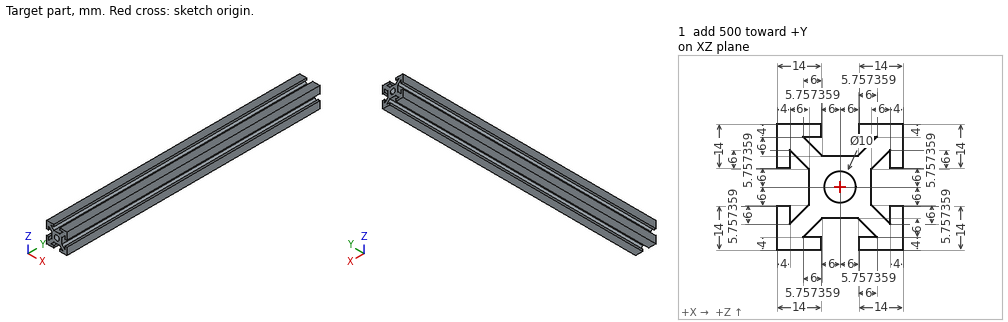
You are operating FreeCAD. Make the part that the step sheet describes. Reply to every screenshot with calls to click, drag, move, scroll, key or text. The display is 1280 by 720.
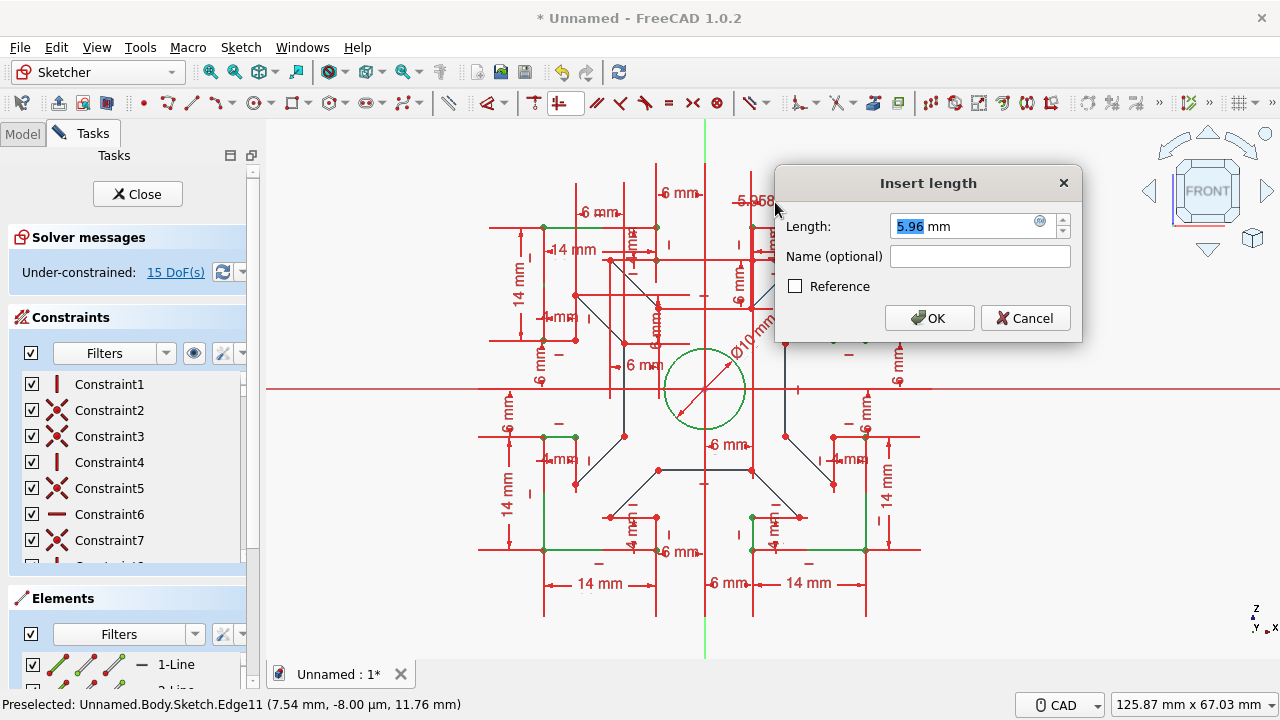
text(6)
key(Return)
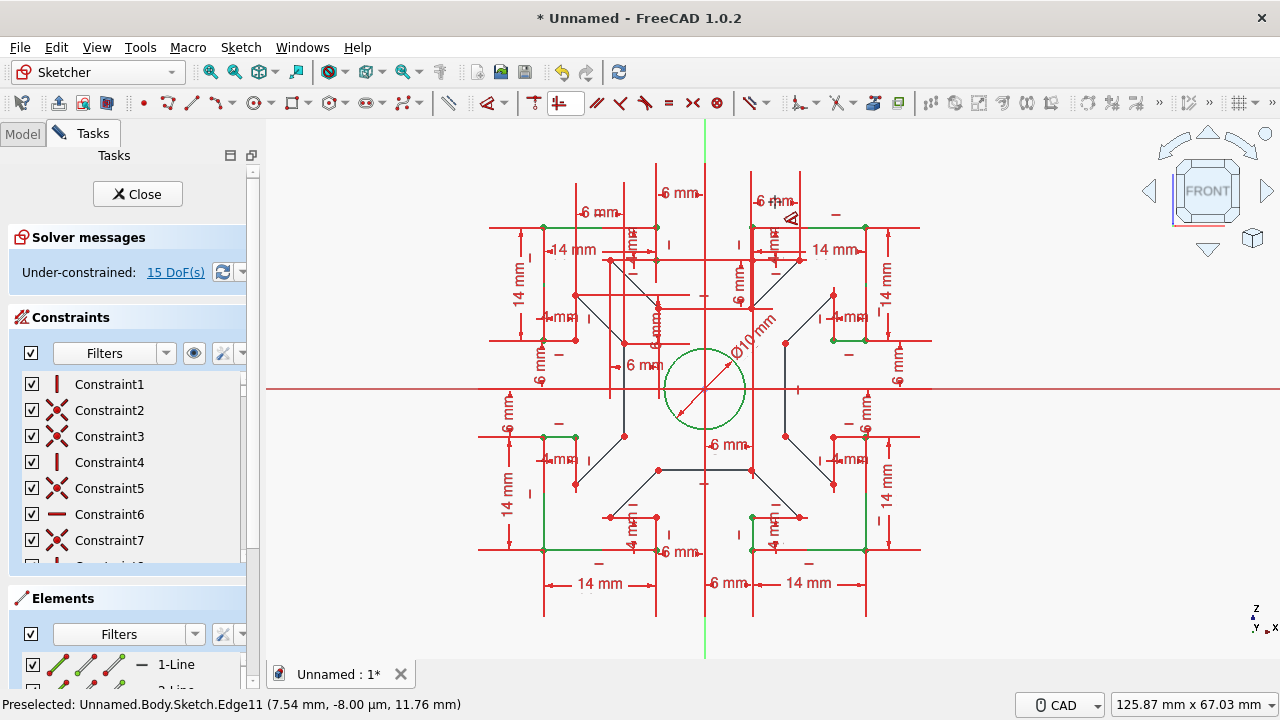
click(819, 310)
click(809, 165)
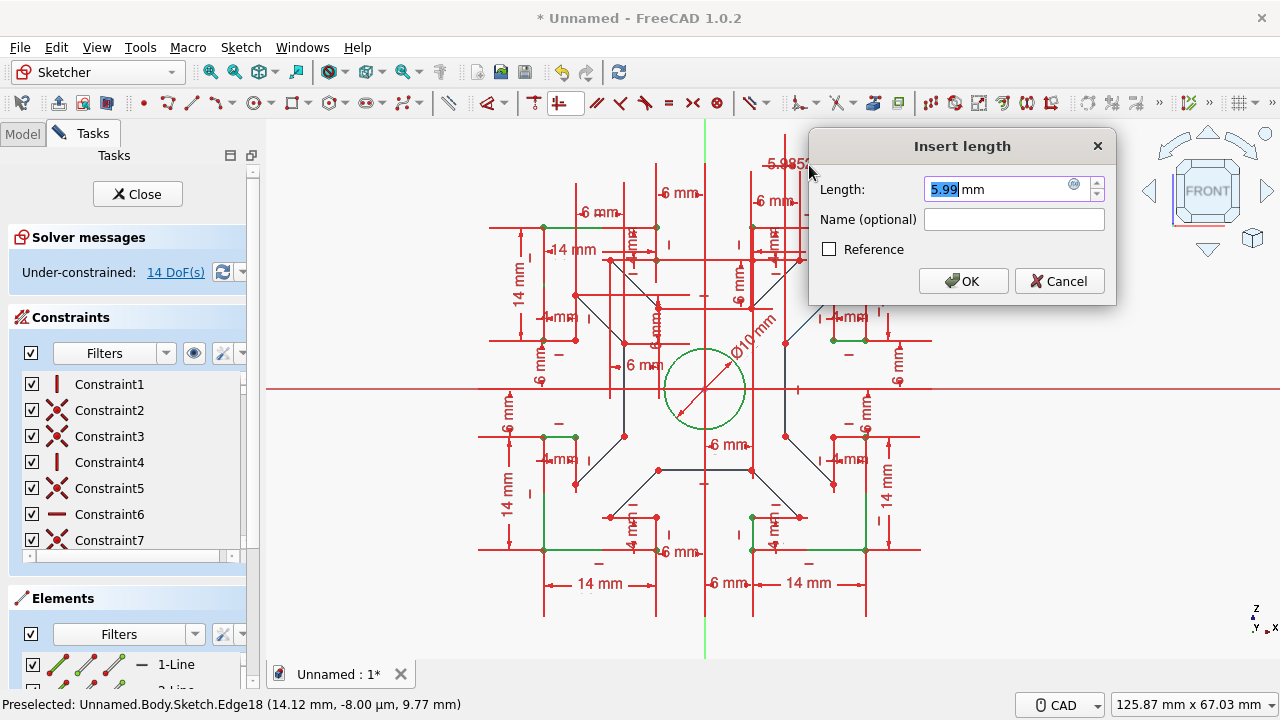
text(6)
key(Return)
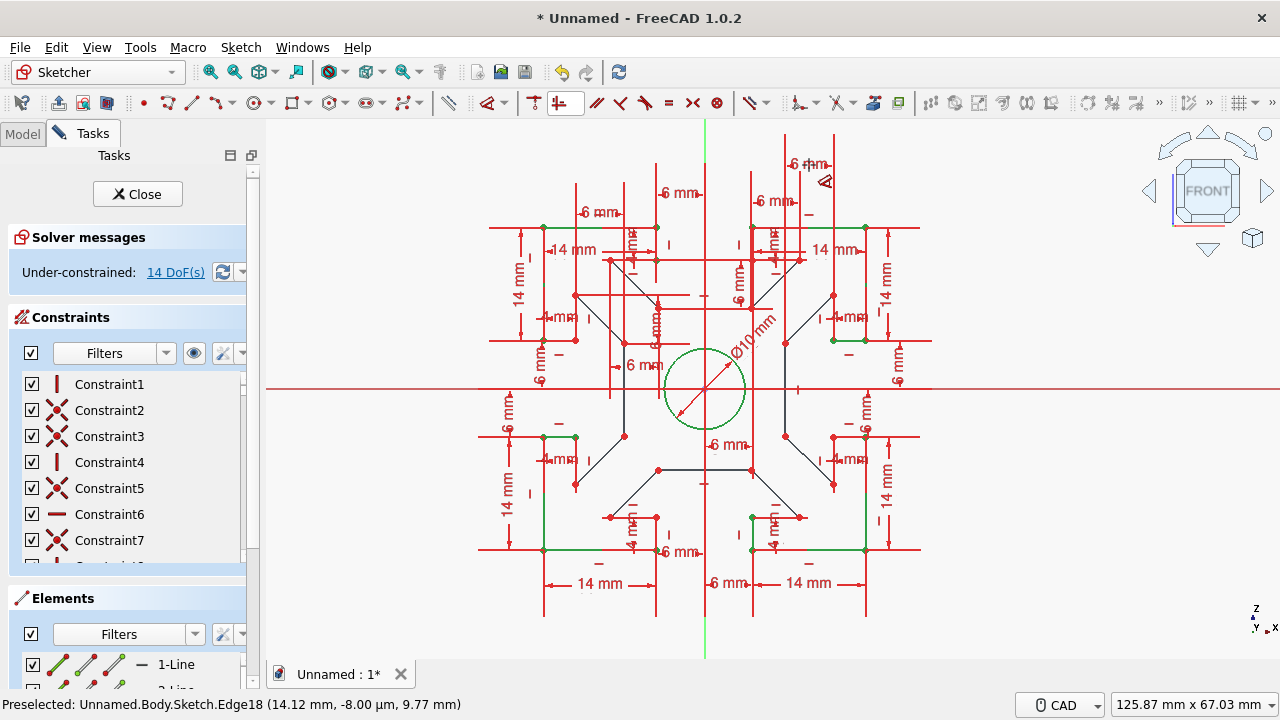
click(819, 310)
click(940, 319)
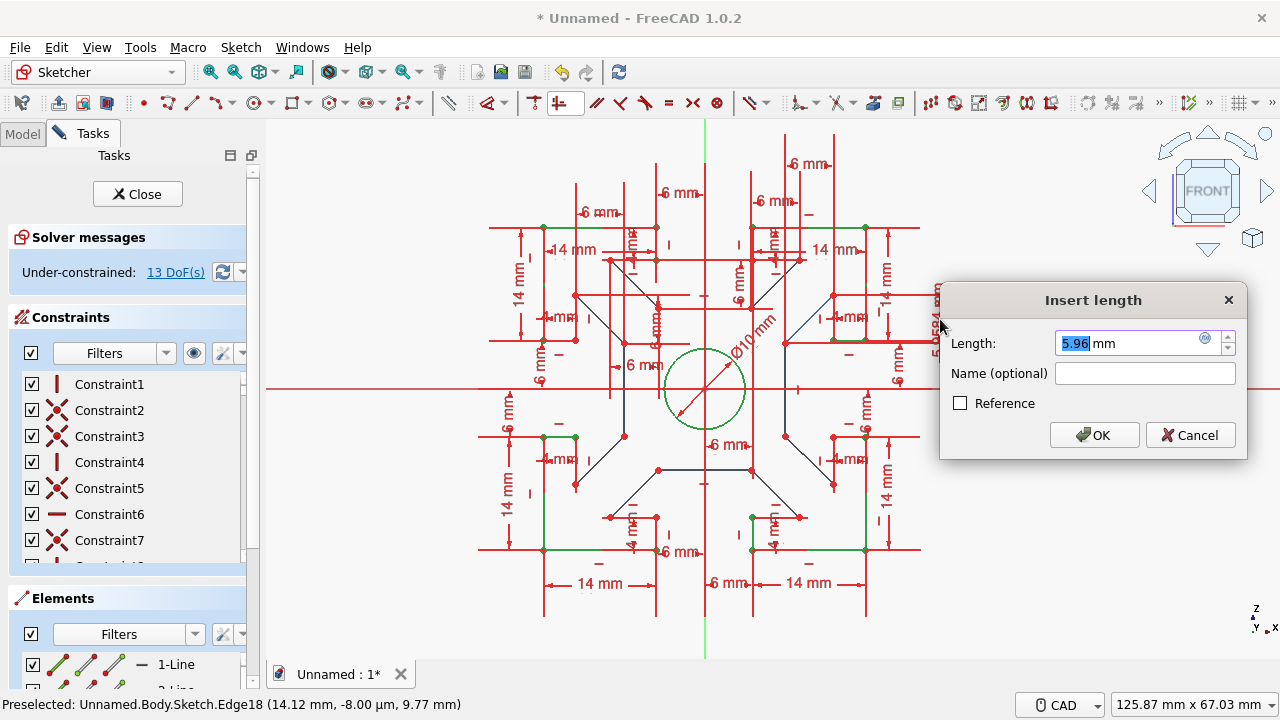
text(6)
key(Return)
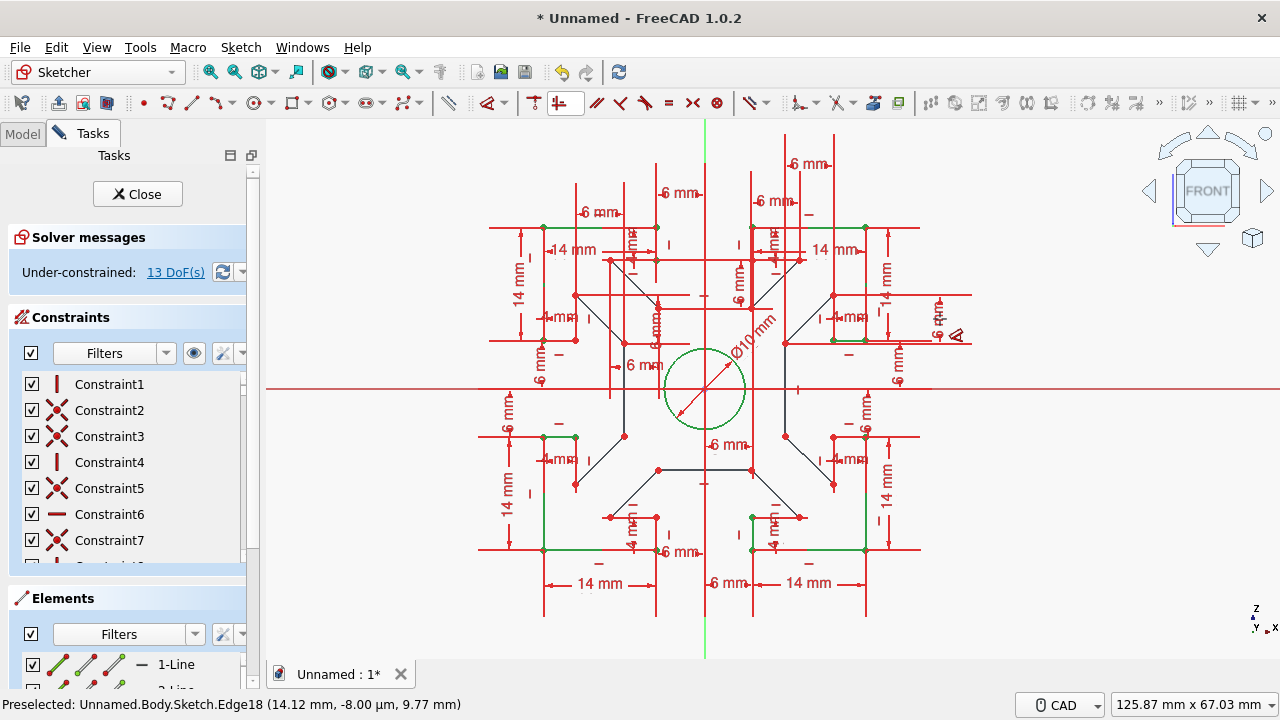
click(800, 451)
click(940, 460)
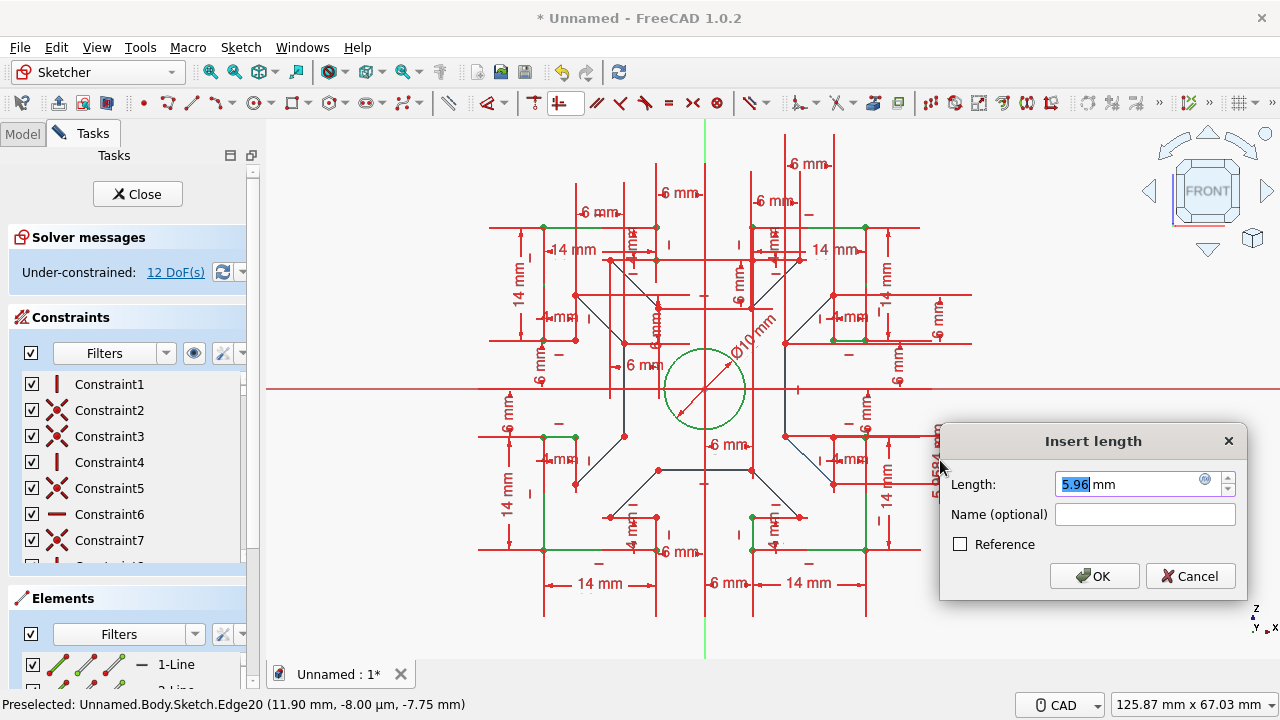
text(6)
key(Return)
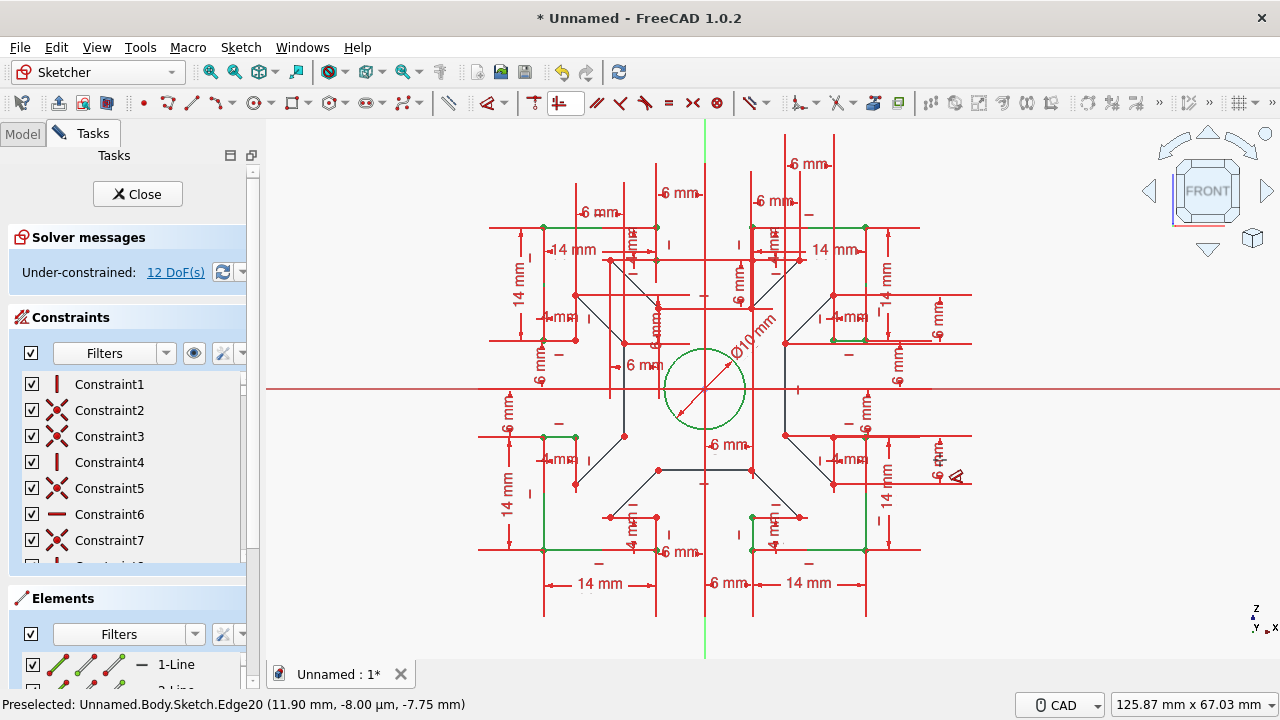
click(785, 504)
click(764, 412)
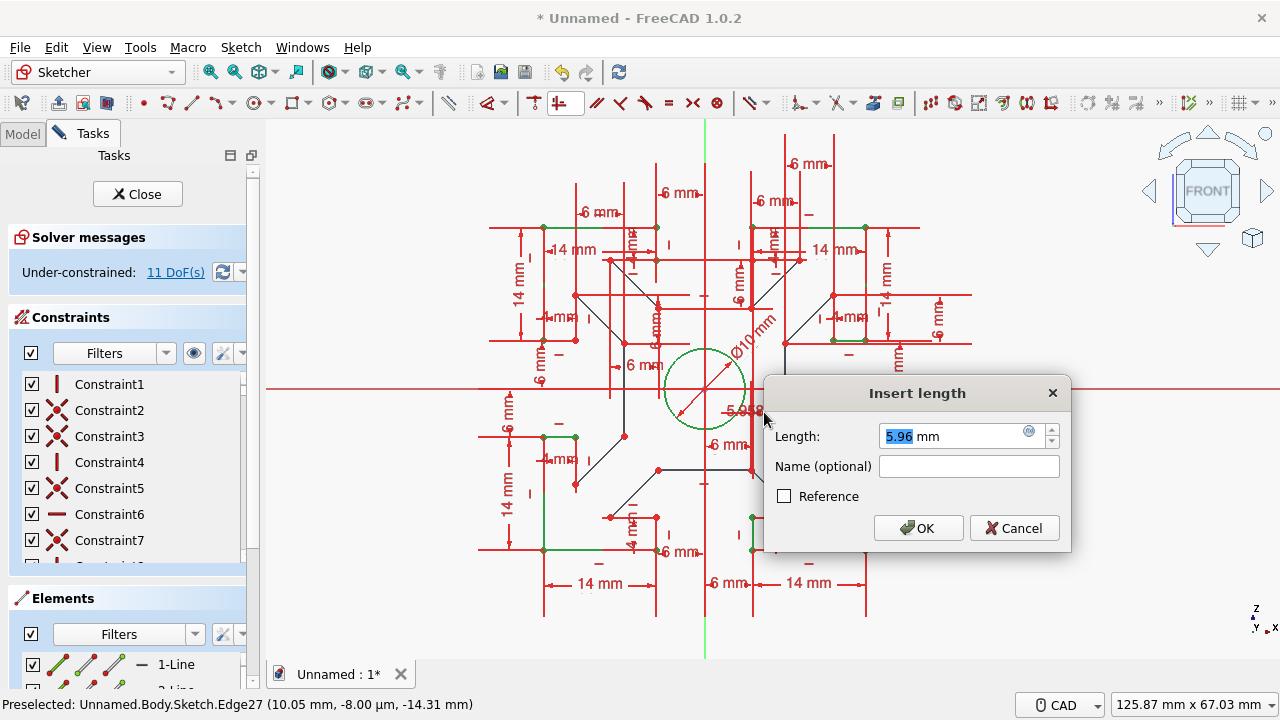
text(6)
key(Return)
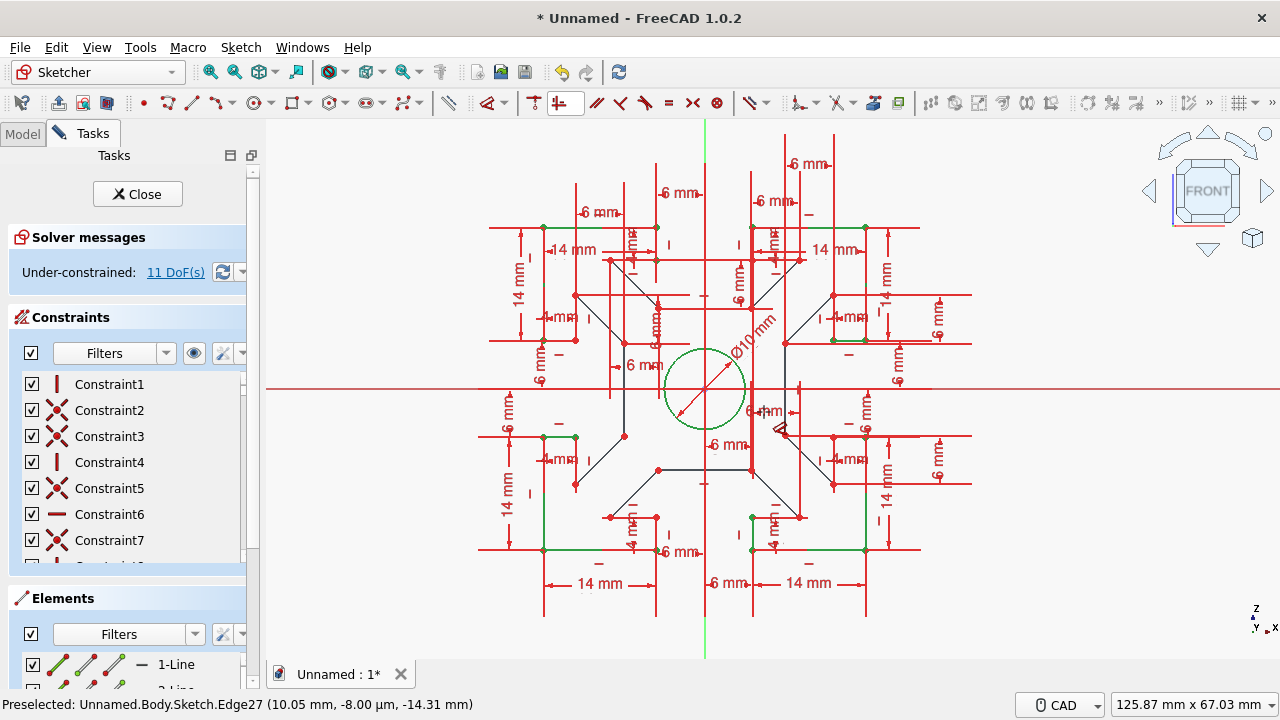
click(785, 504)
click(834, 511)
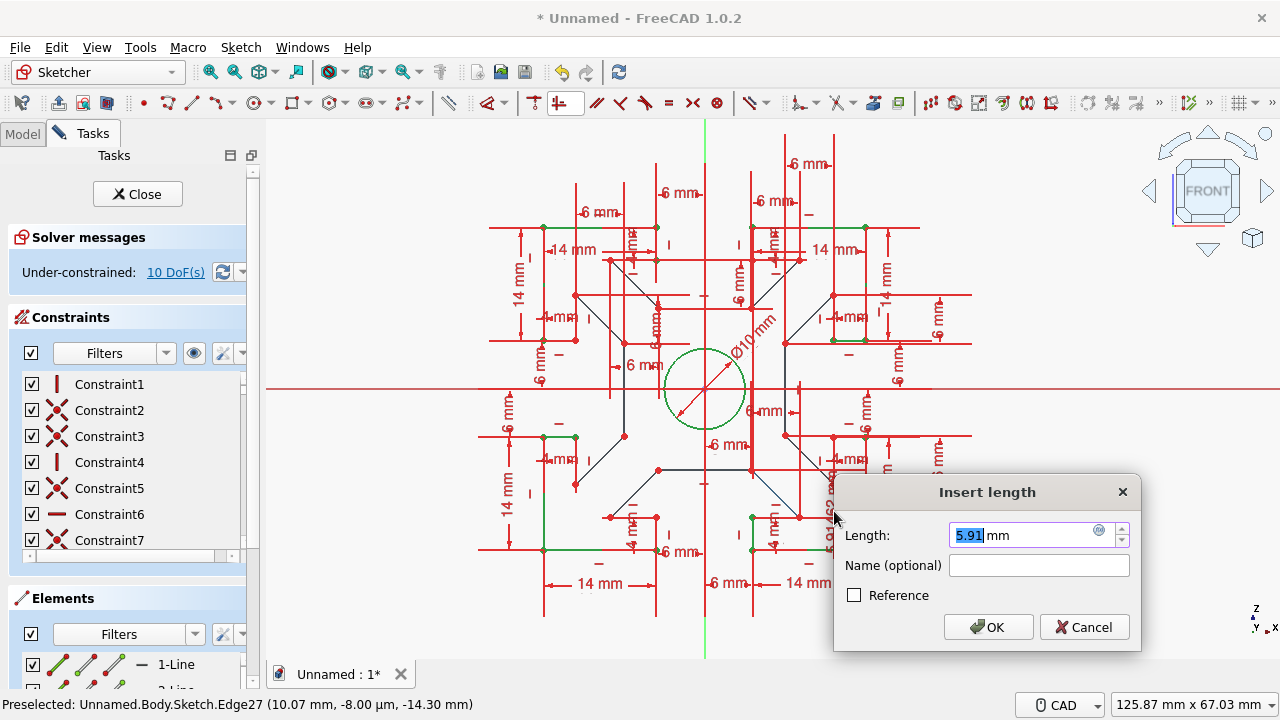
text(6)
key(Return)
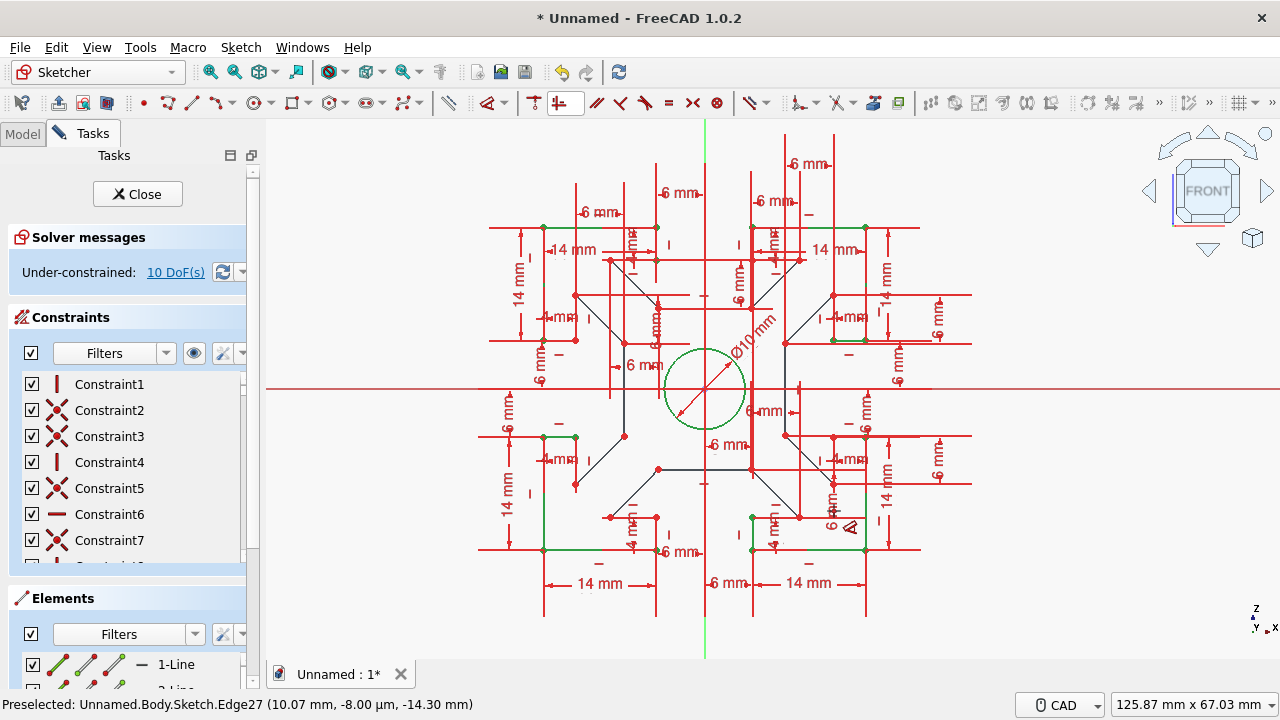
click(644, 484)
click(645, 436)